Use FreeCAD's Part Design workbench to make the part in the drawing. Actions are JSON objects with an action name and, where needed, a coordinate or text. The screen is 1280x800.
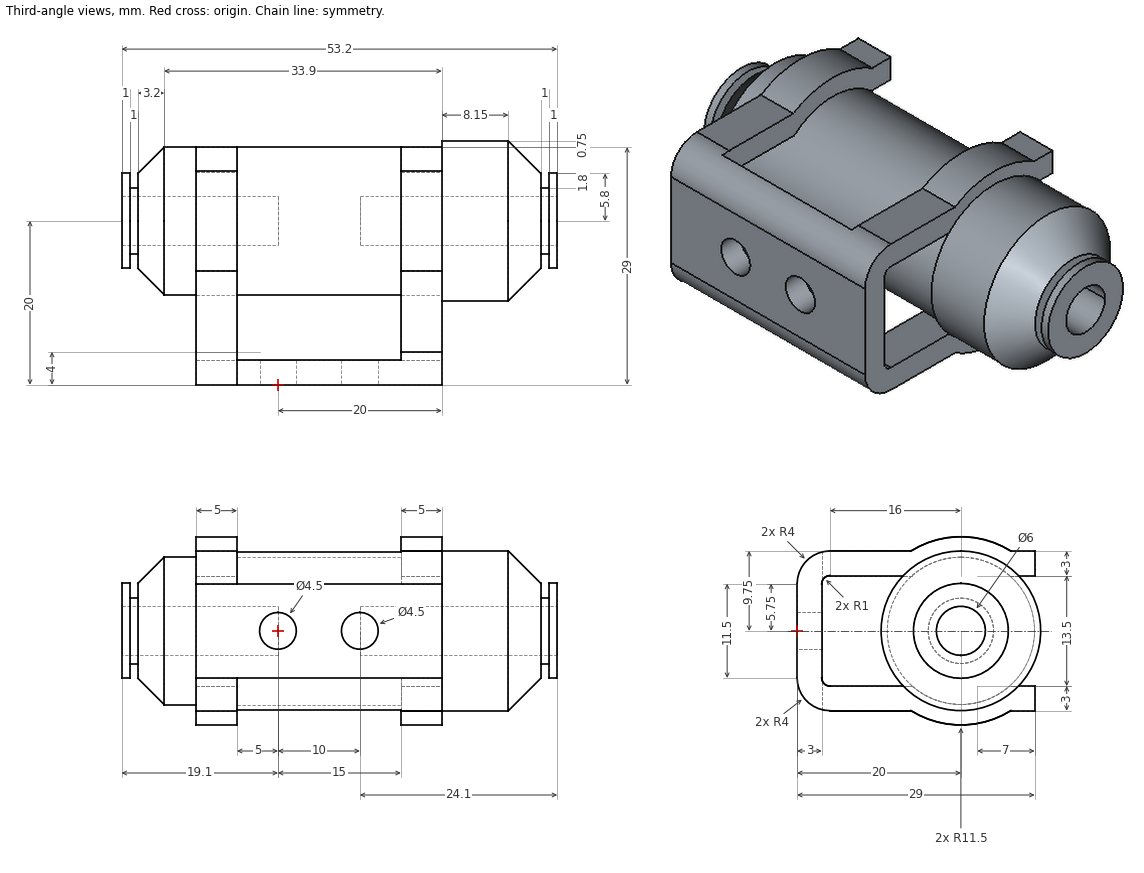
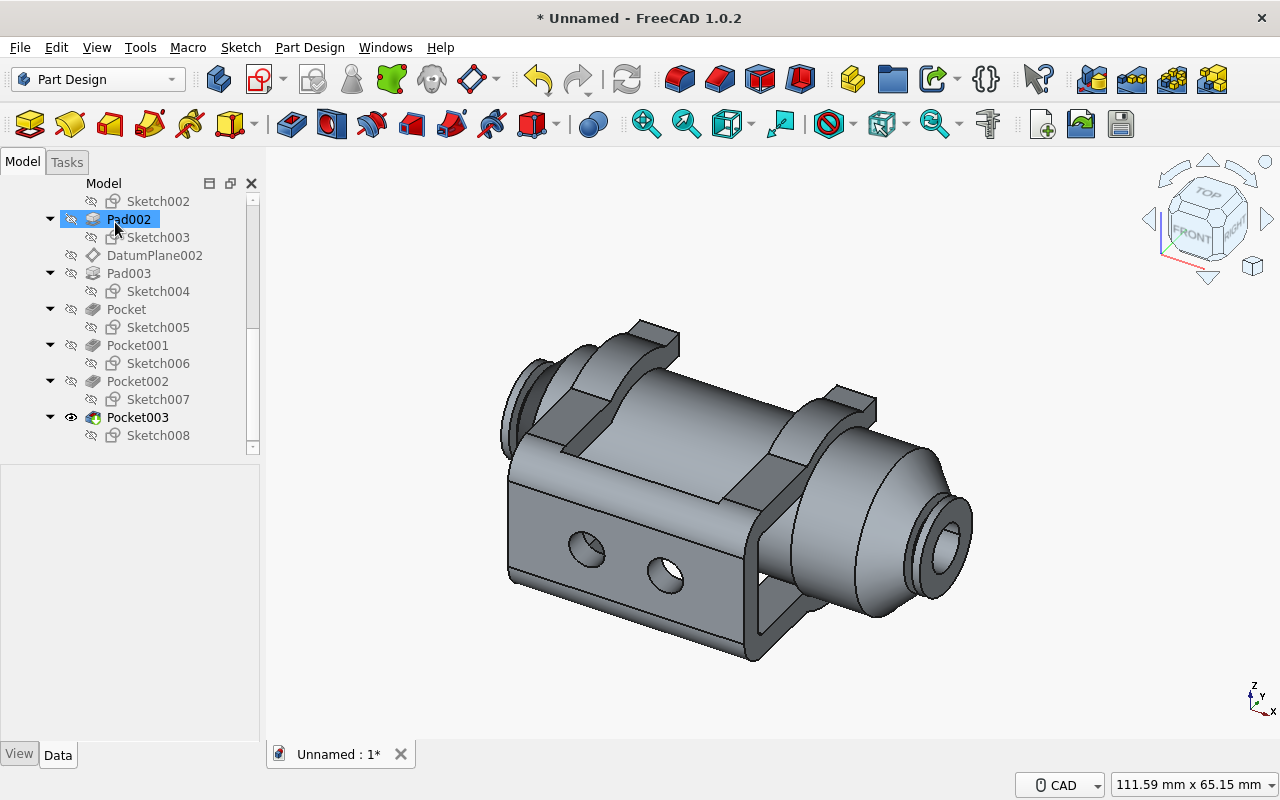
{"action": "key", "text": "0"}